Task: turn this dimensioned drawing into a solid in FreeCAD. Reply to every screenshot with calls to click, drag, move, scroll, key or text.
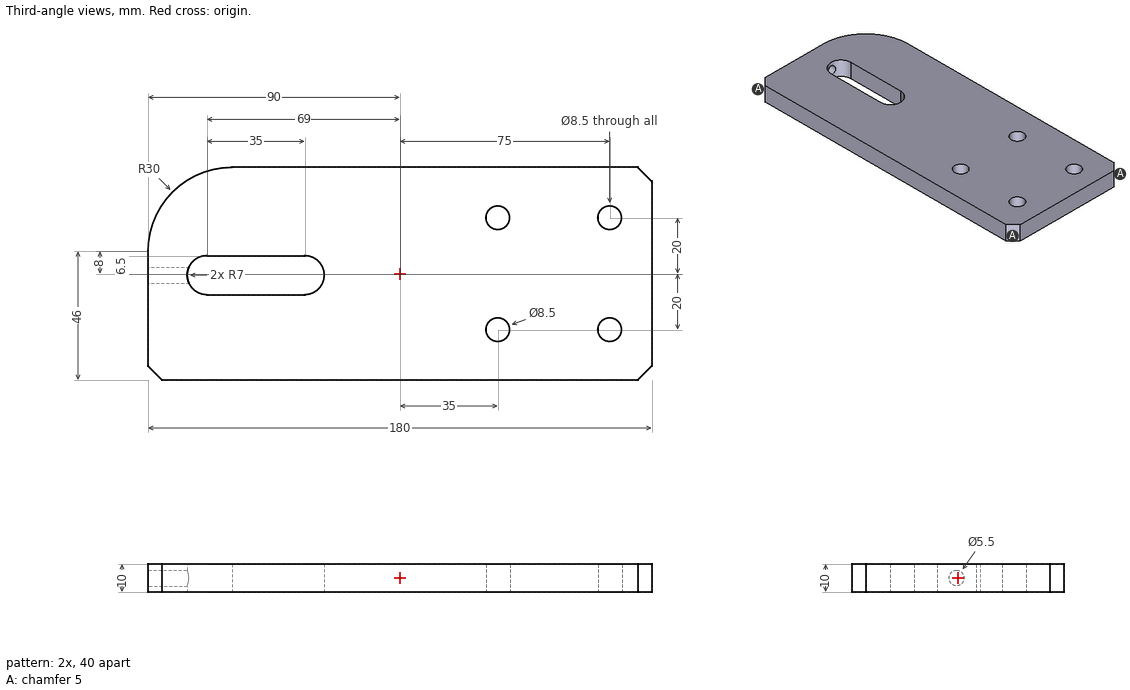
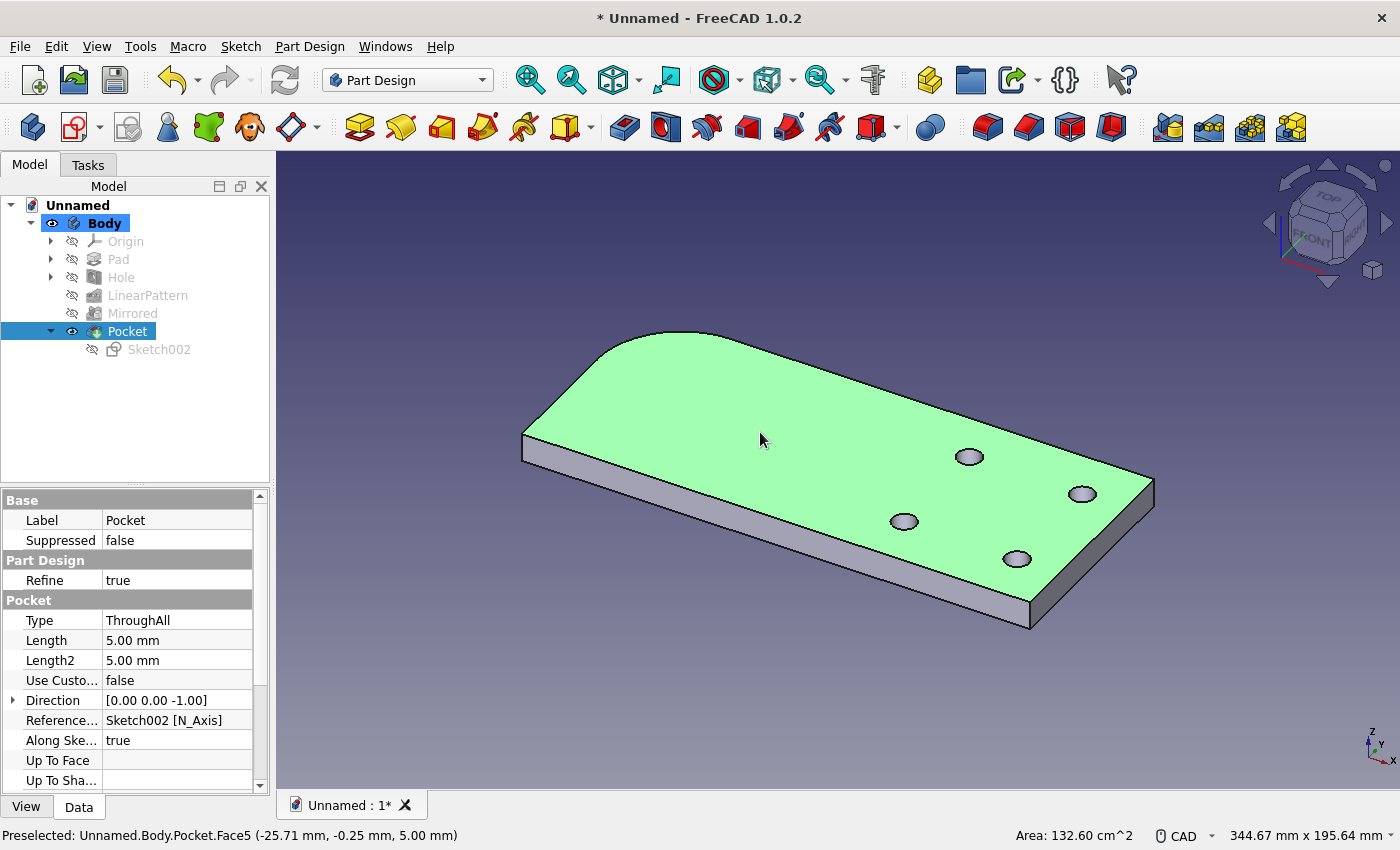
click(74, 128)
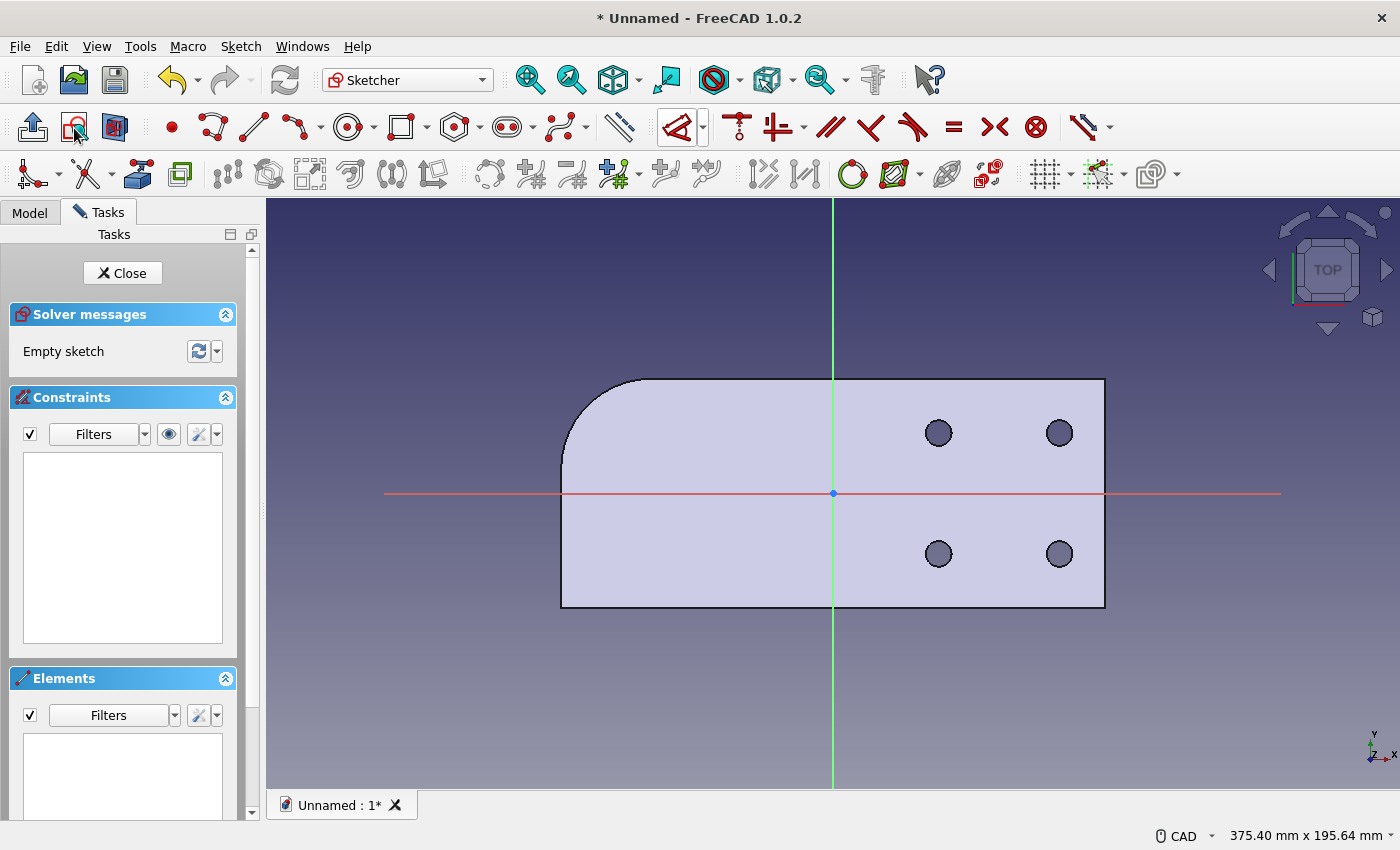
scroll(691, 496, up, 5)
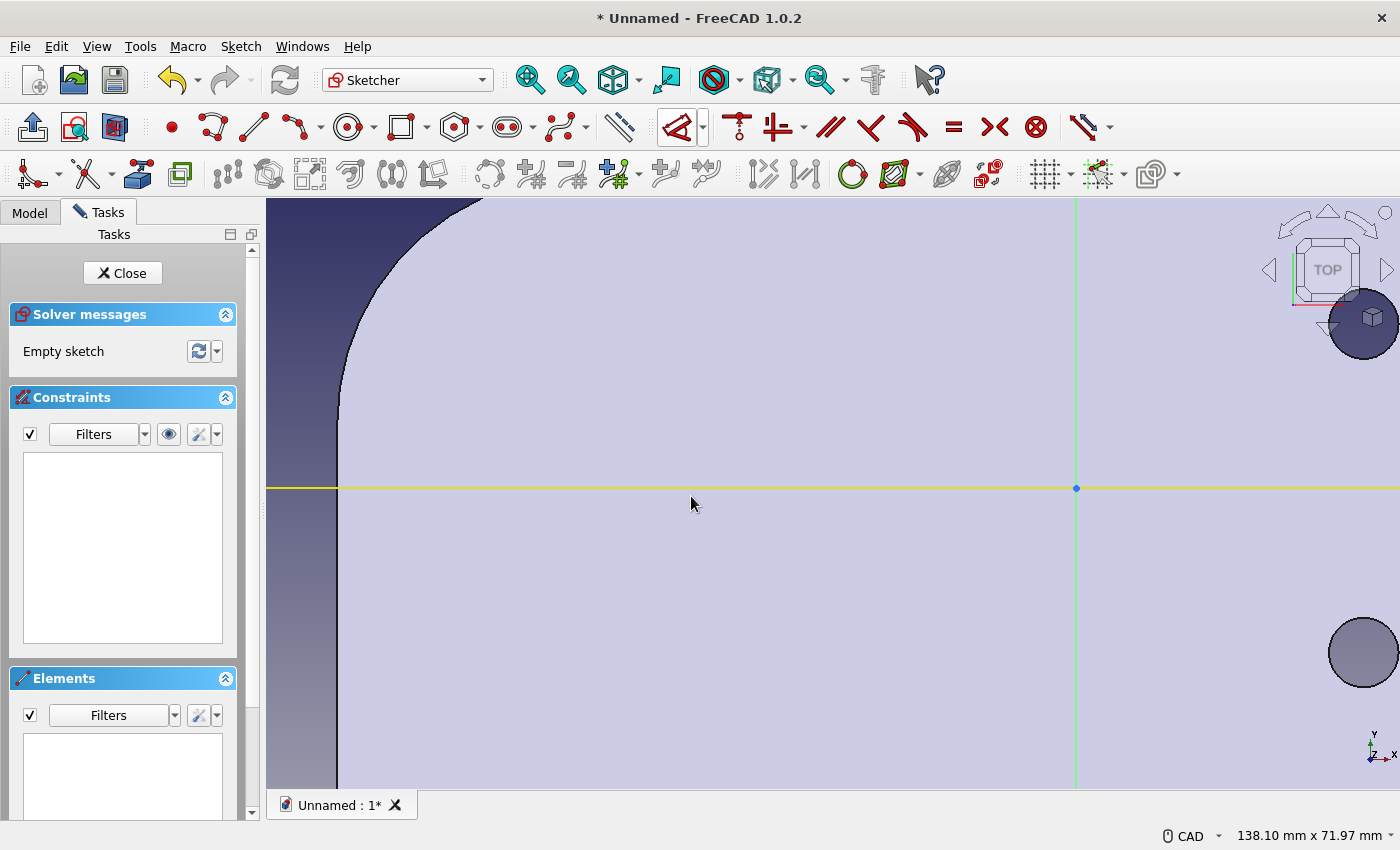
key(g)
key(s)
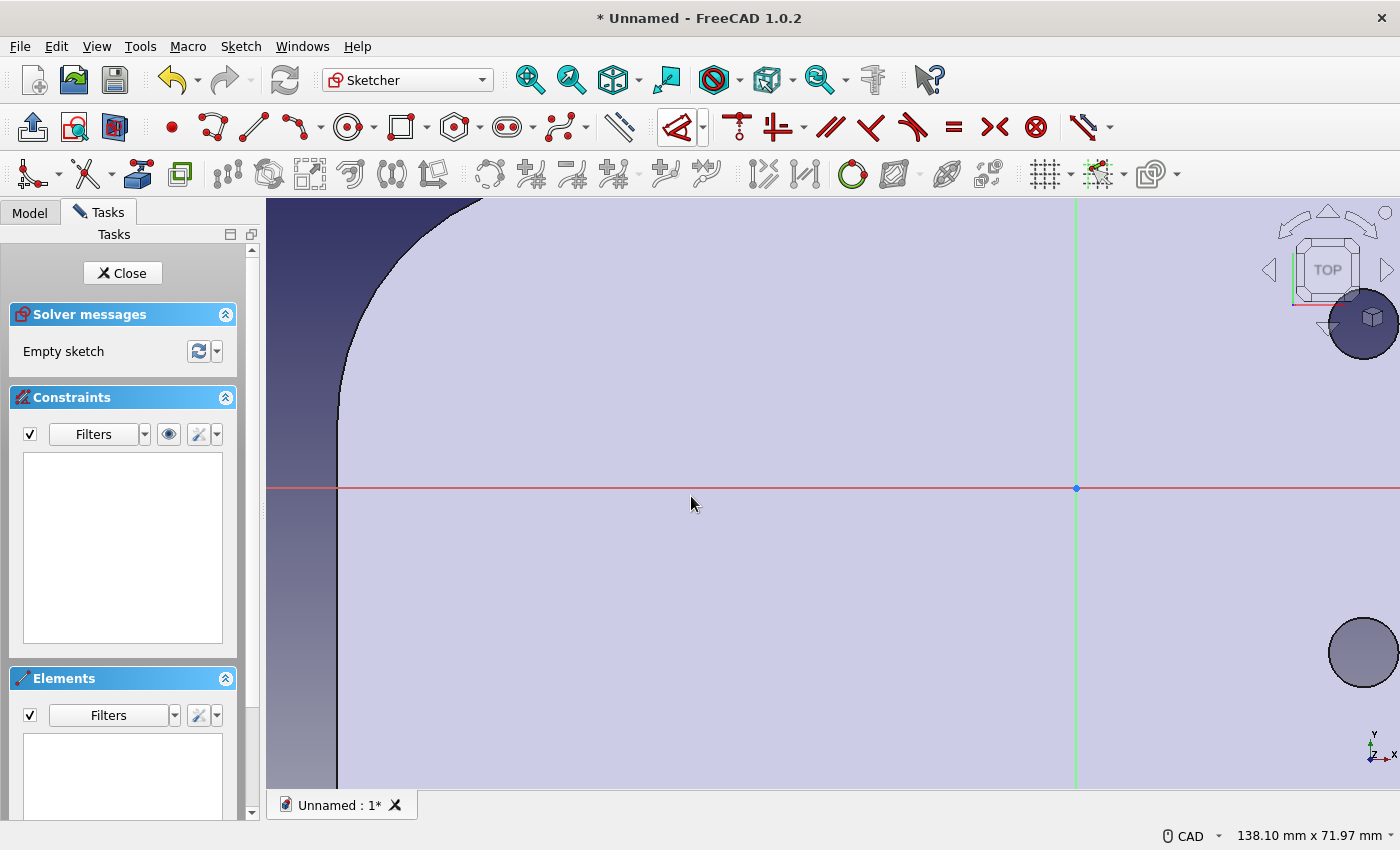
scroll(510, 492, up, 7)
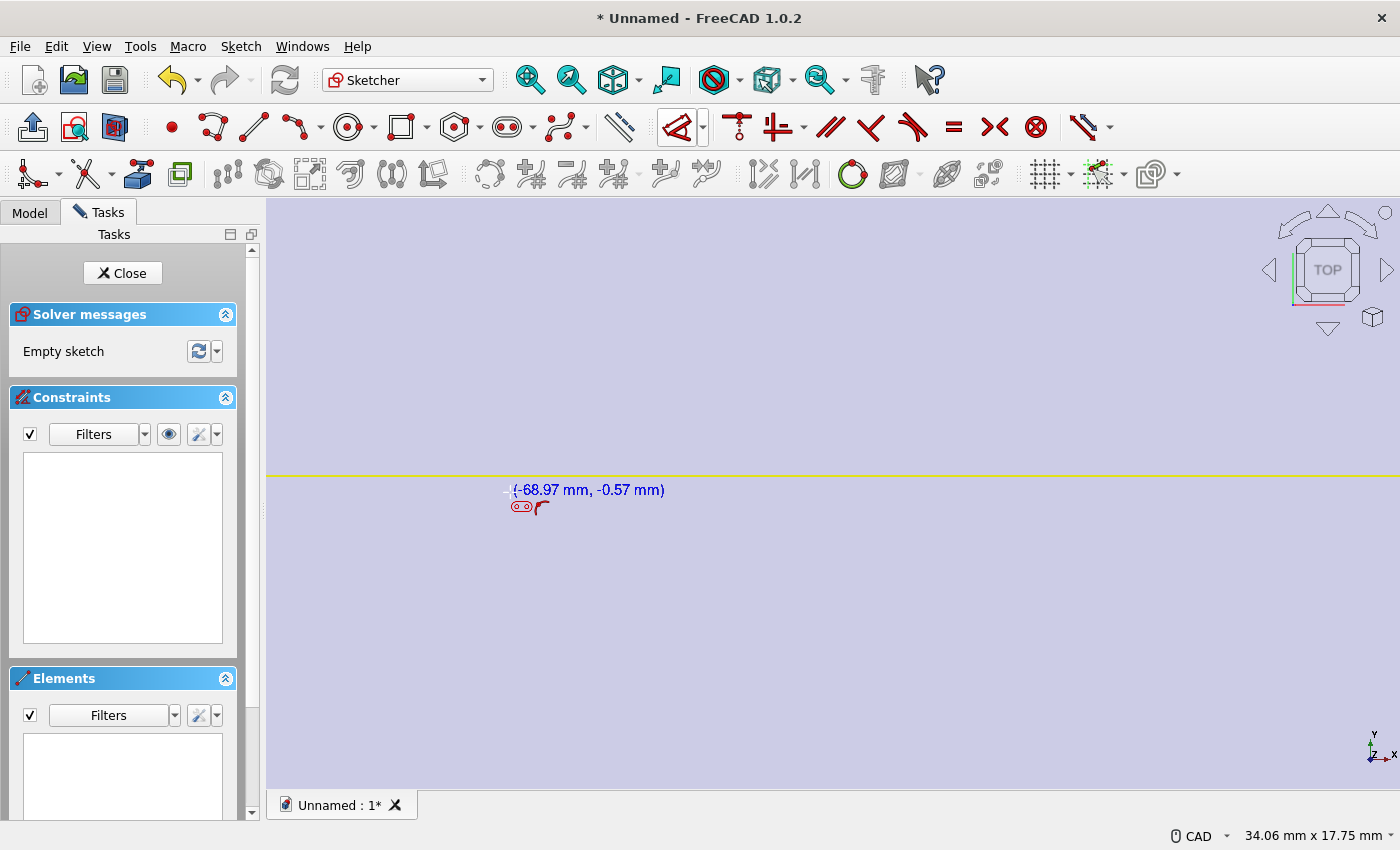
click(508, 492)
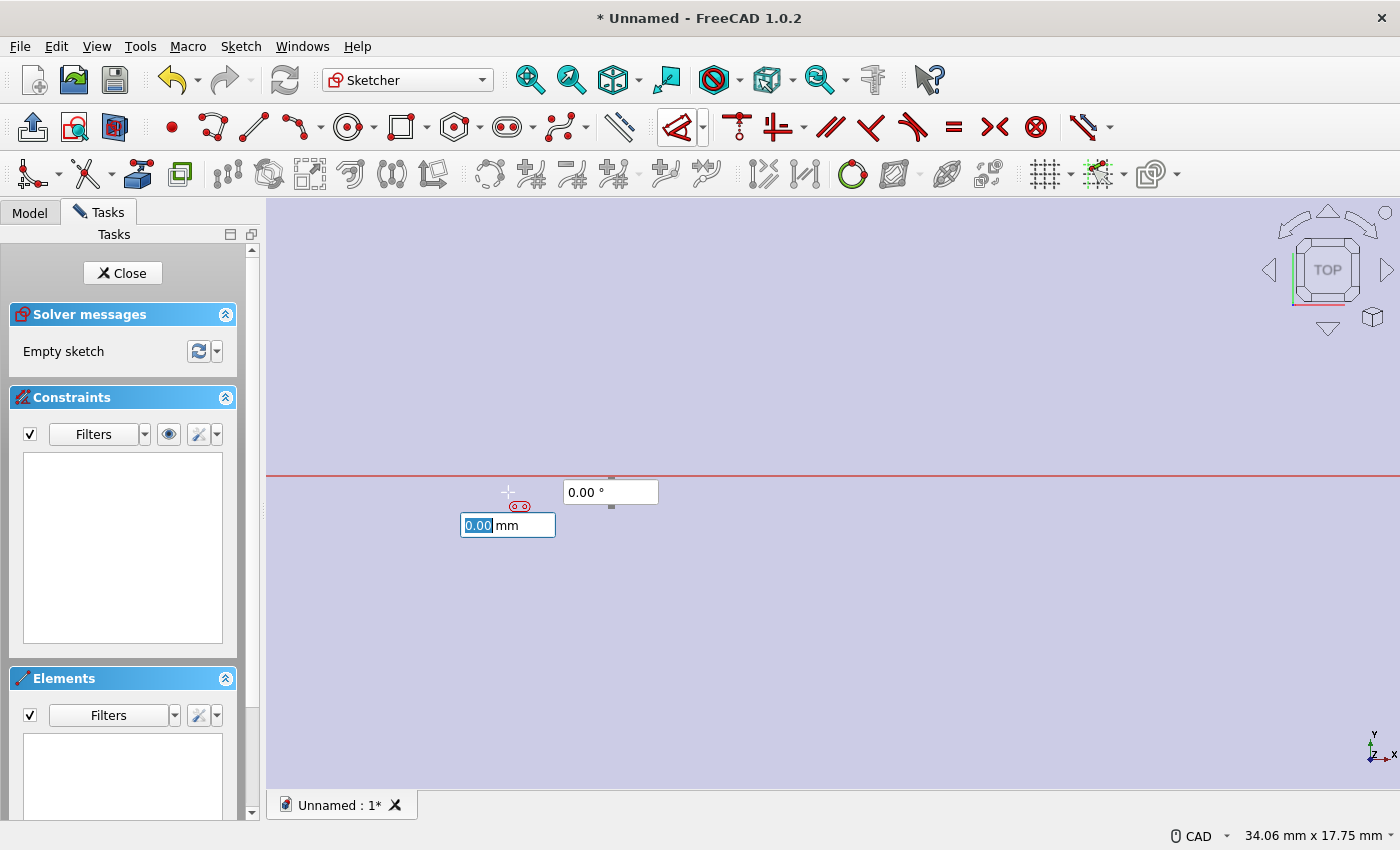
scroll(510, 494, down, 7)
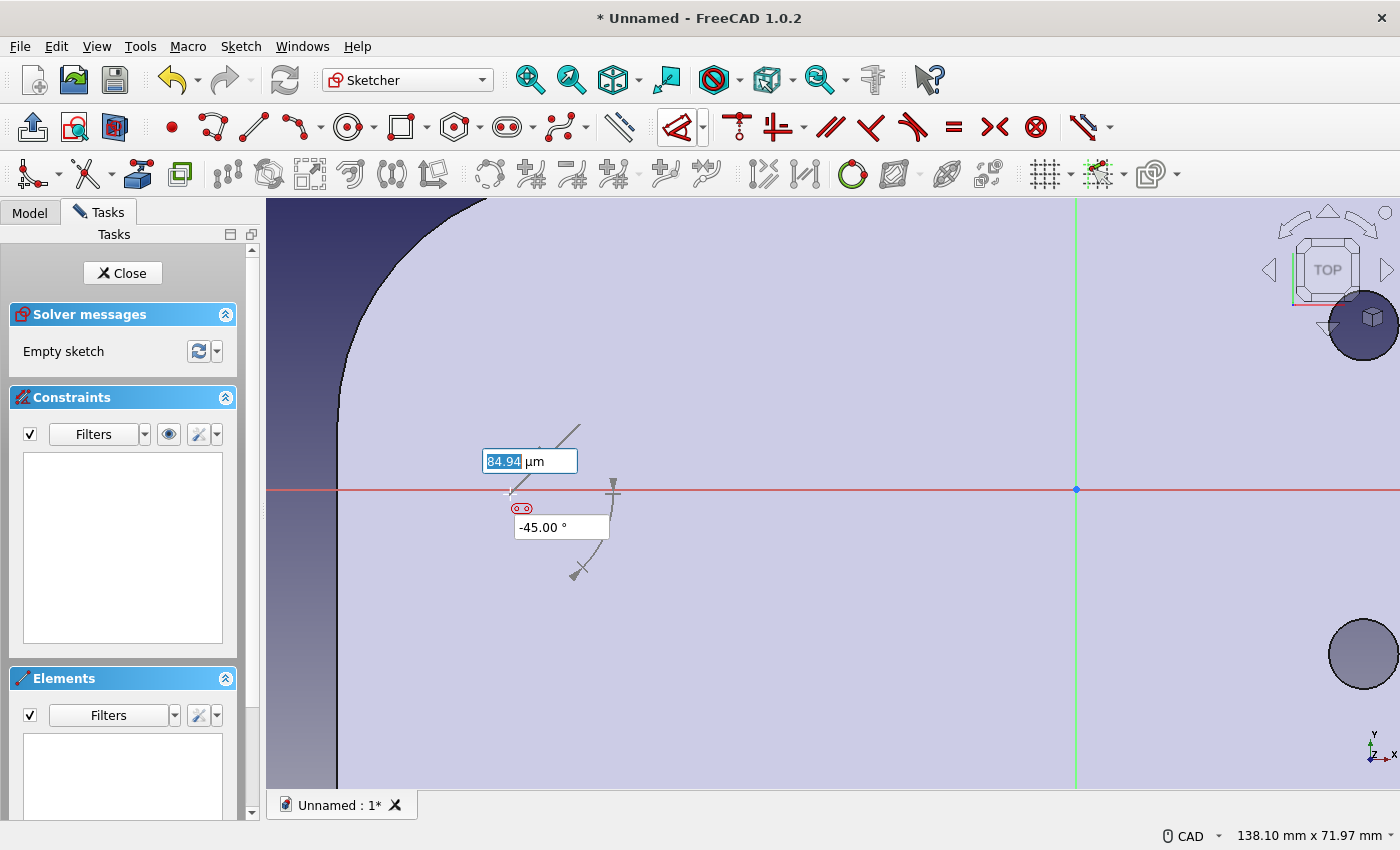
scroll(797, 494, up, 7)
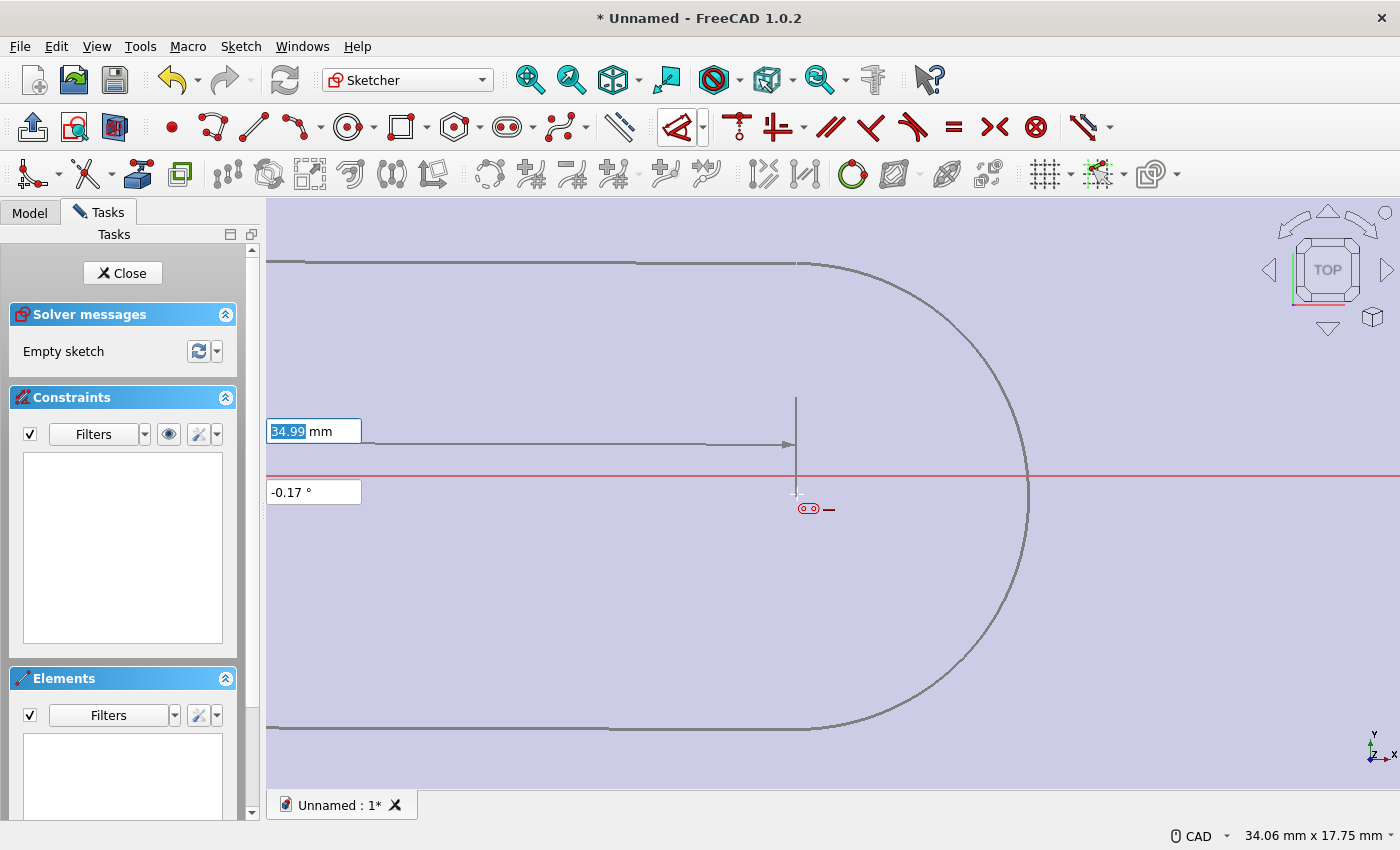
click(796, 492)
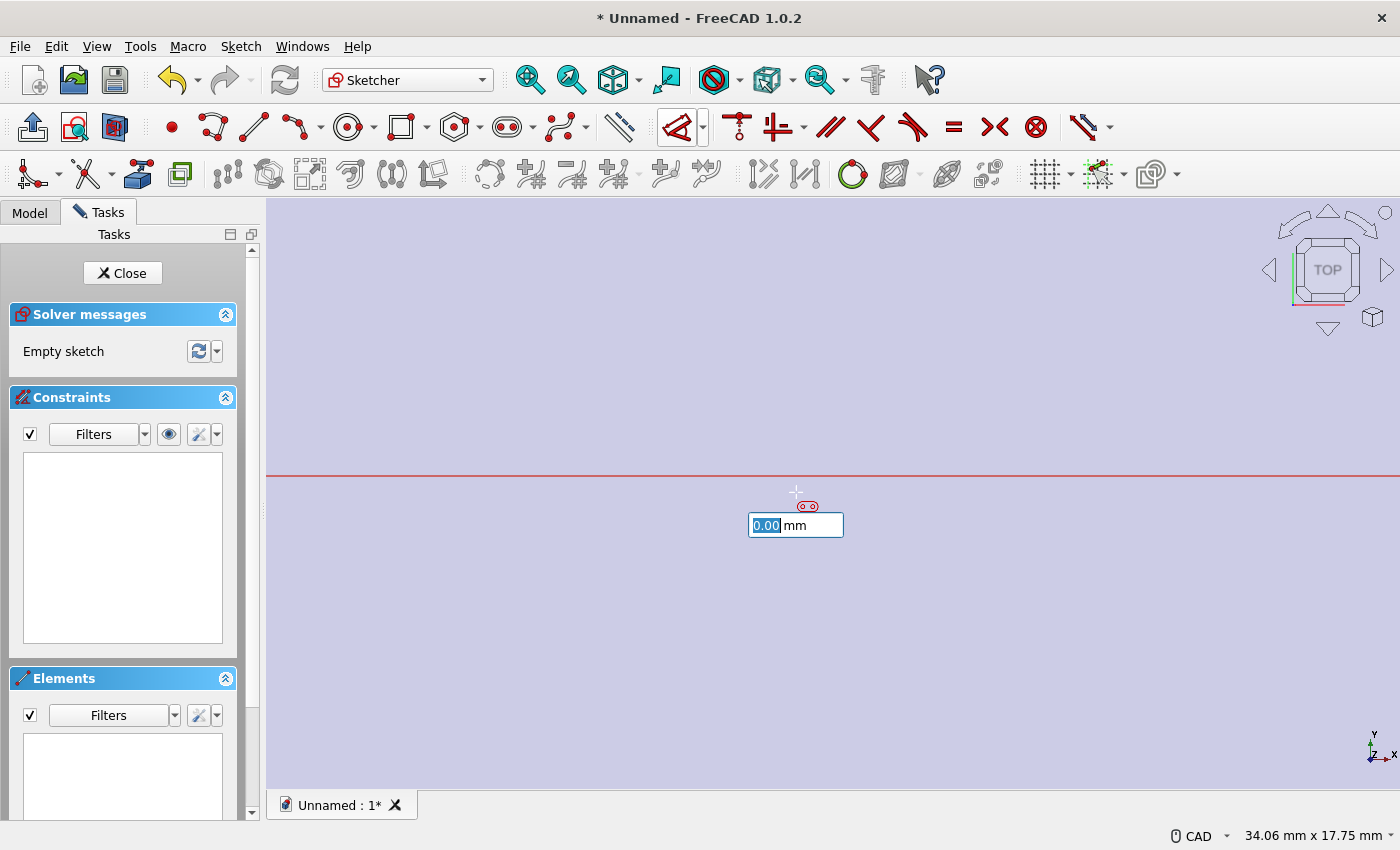
scroll(798, 494, down, 7)